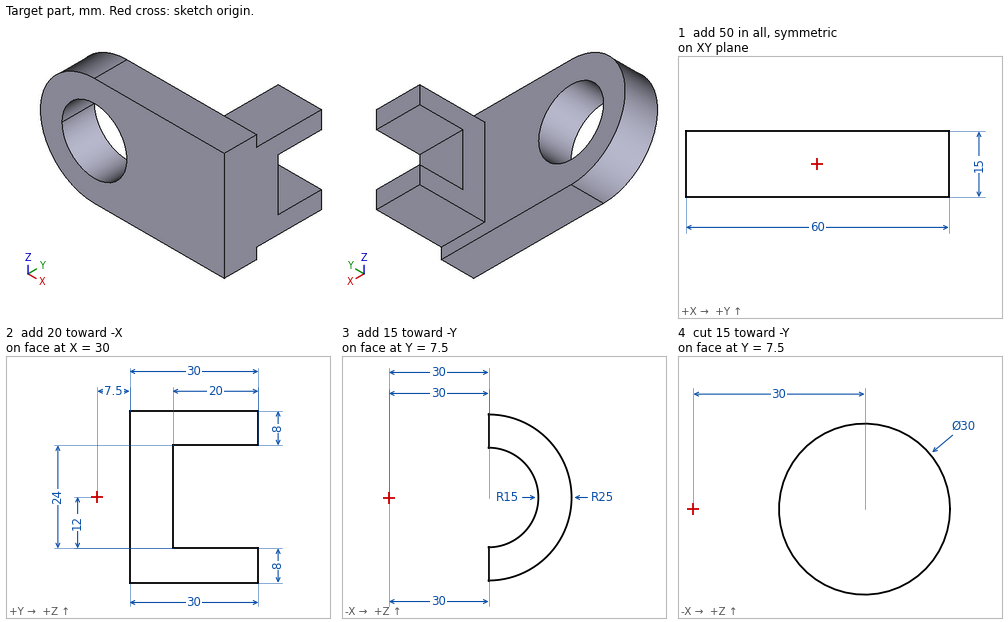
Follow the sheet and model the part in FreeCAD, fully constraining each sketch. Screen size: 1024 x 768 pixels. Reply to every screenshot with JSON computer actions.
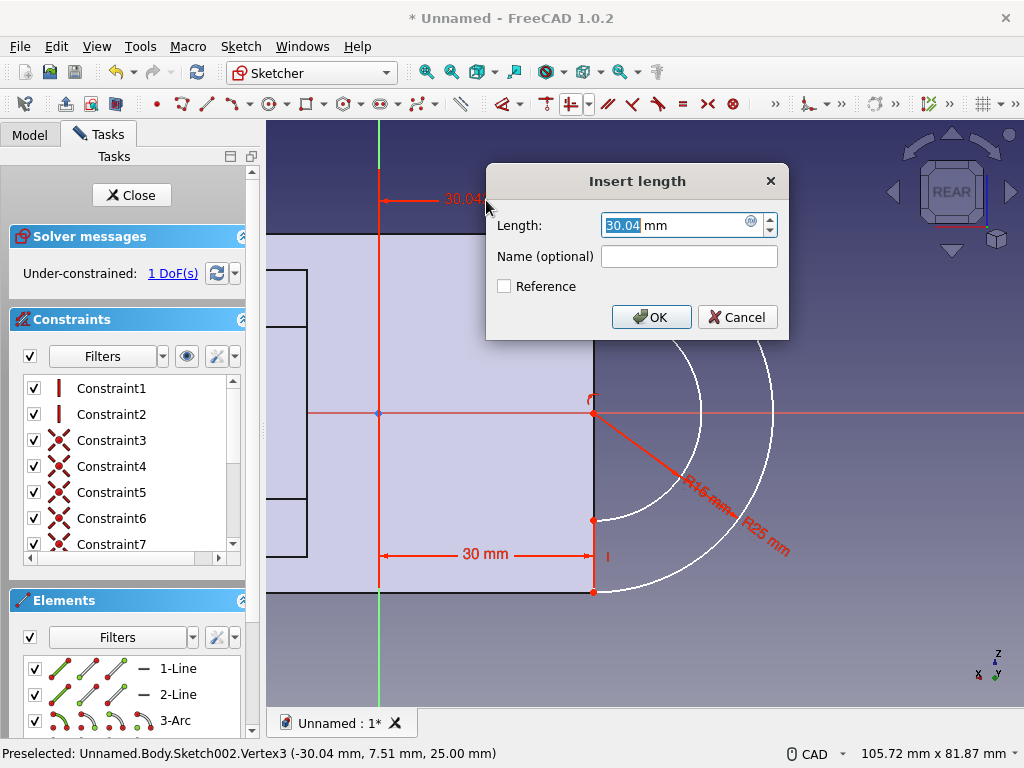
{"action": "type", "text": "30"}
{"action": "key", "text": "Return"}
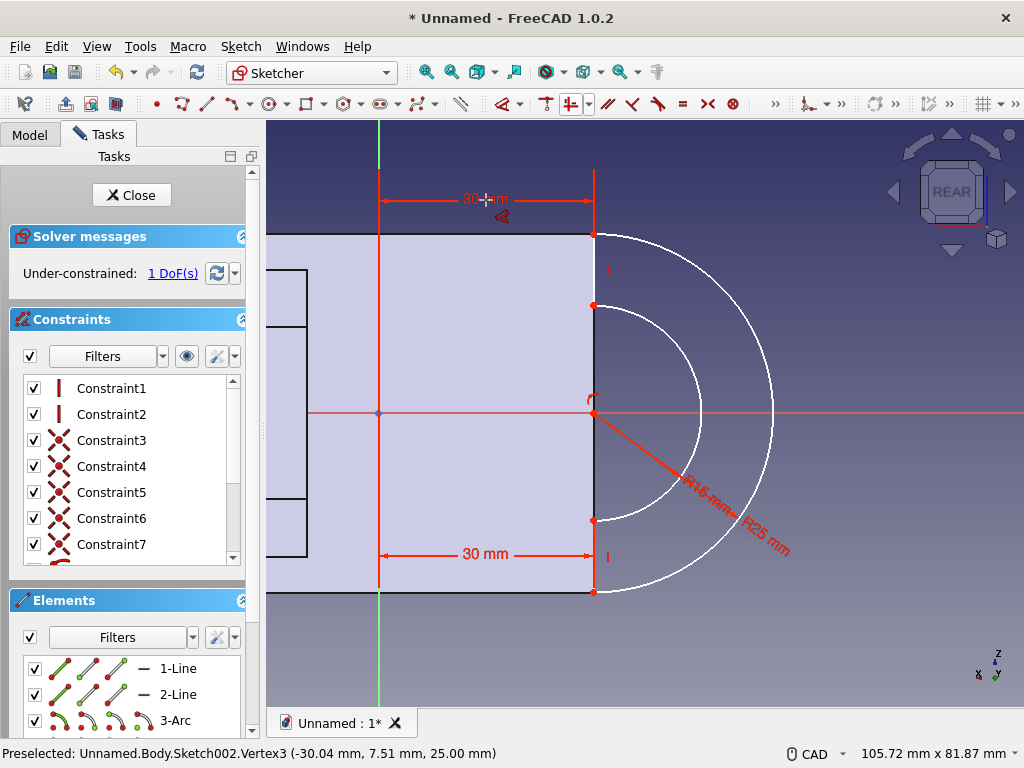
{"action": "left_click", "coordinate": [594, 413]}
{"action": "left_click", "coordinate": [486, 447]}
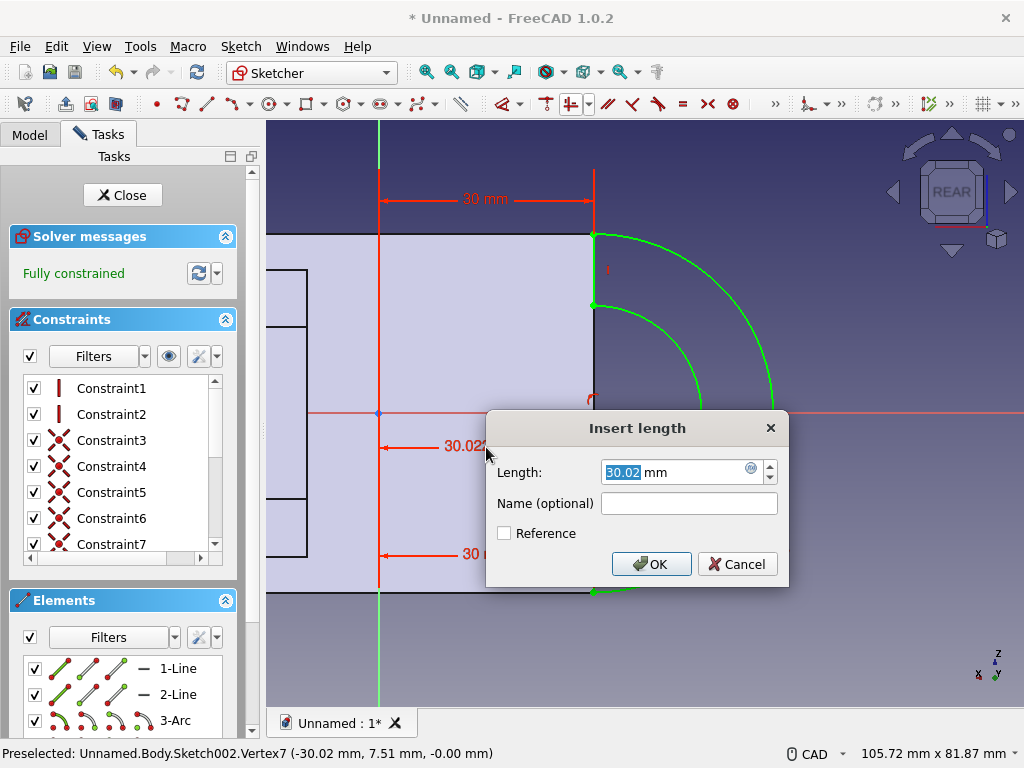
{"action": "type", "text": "30"}
{"action": "key", "text": "Return"}
{"action": "key", "text": "Escape"}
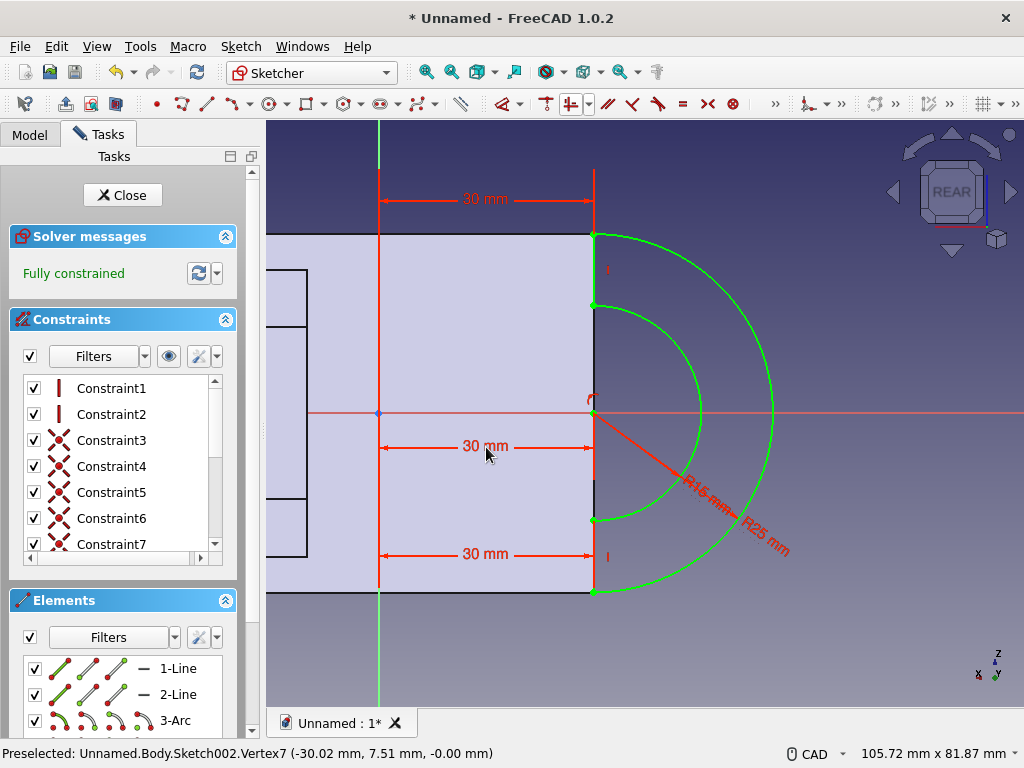
{"action": "left_click", "coordinate": [123, 195]}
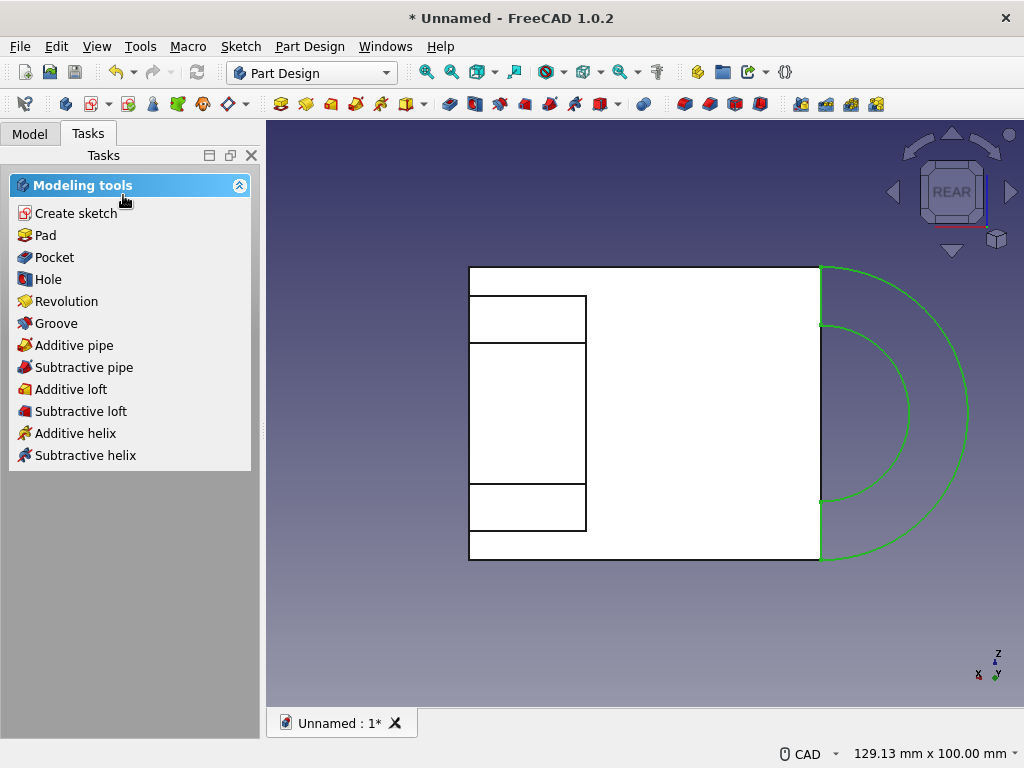
{"action": "left_click", "coordinate": [281, 104]}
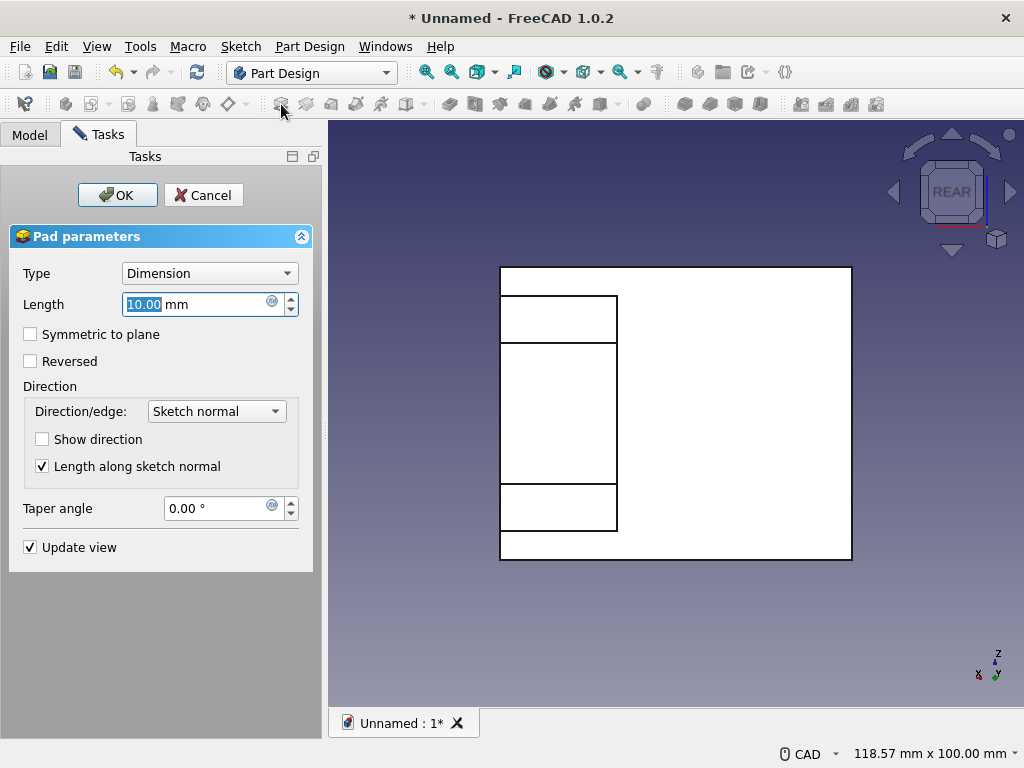
{"action": "type", "text": "15"}
{"action": "key", "text": "Tab"}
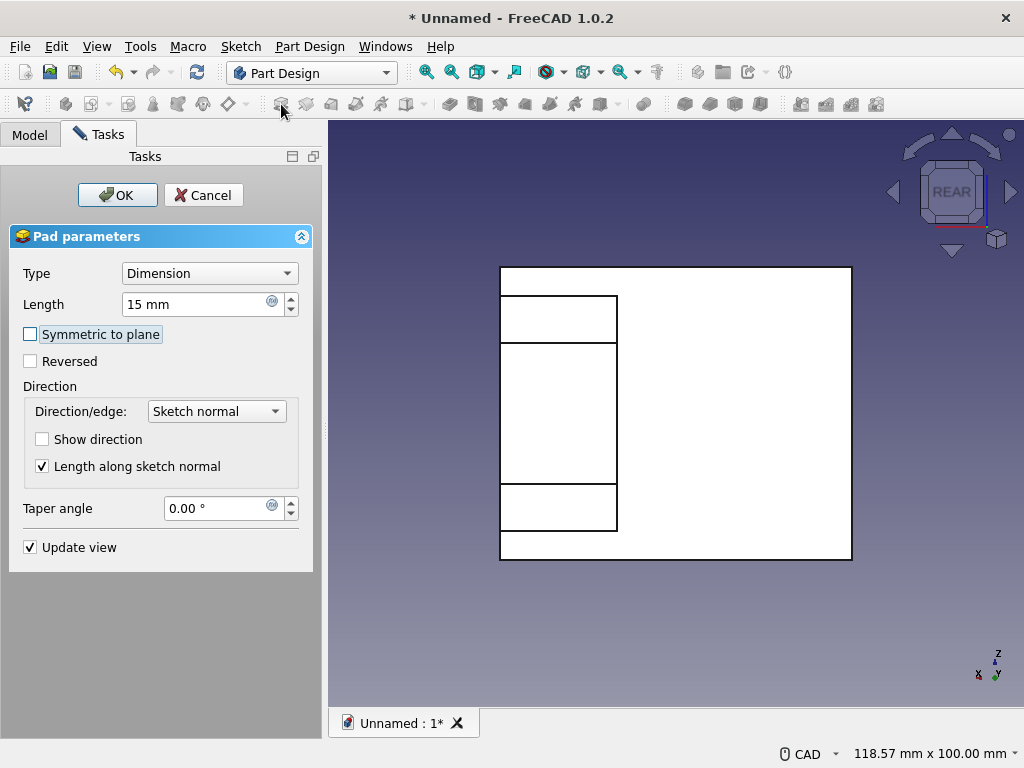
{"action": "left_click", "coordinate": [31, 361]}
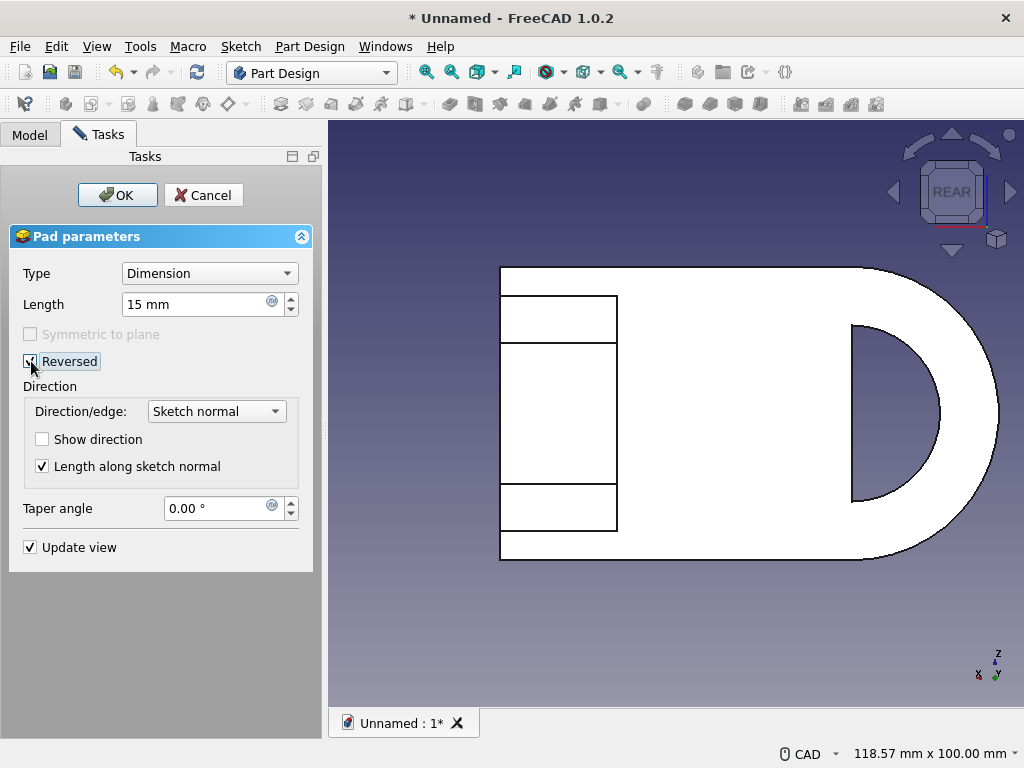
{"action": "left_click", "coordinate": [118, 195]}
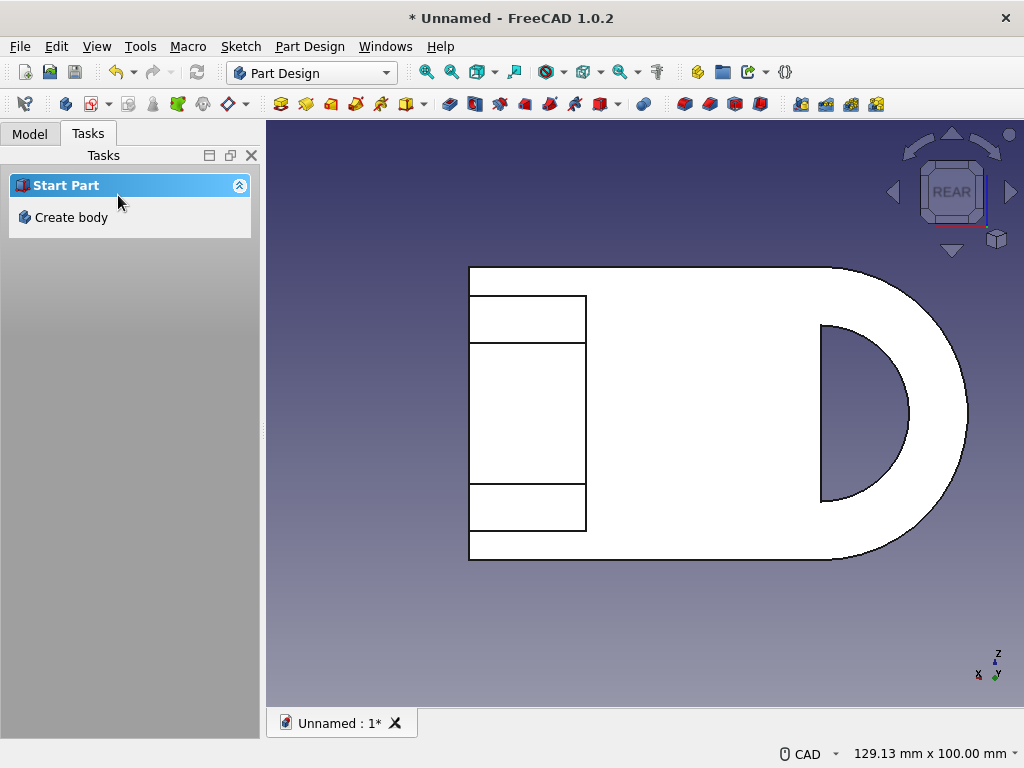
{"action": "left_click", "coordinate": [718, 371]}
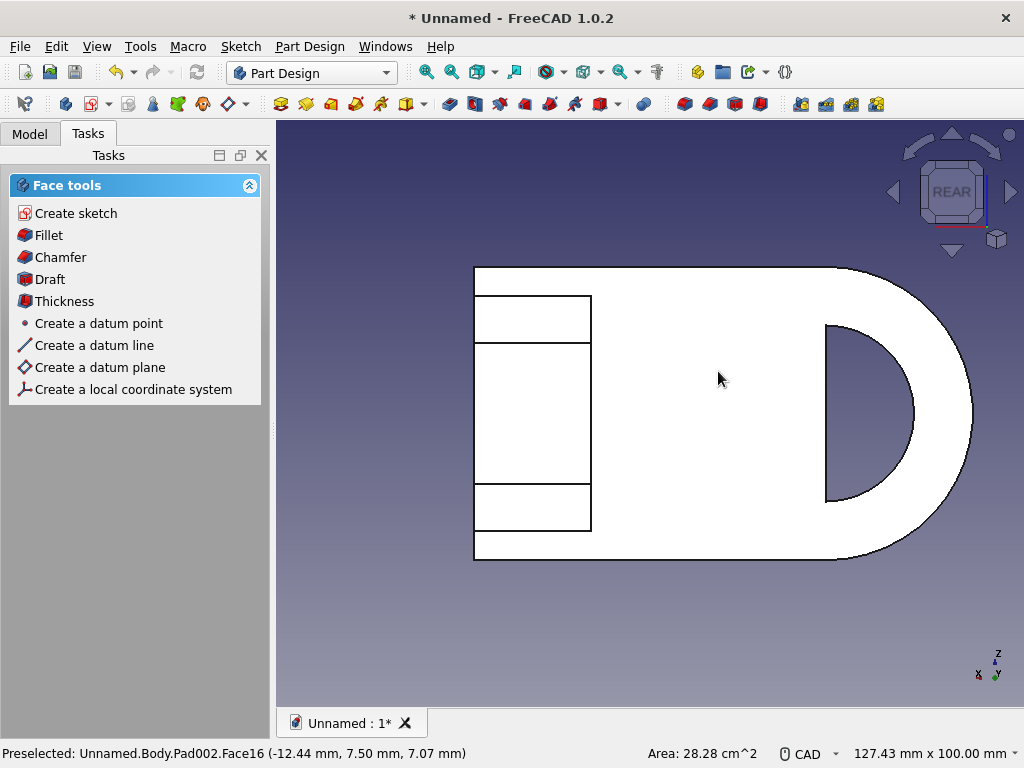
{"action": "left_click", "coordinate": [90, 104]}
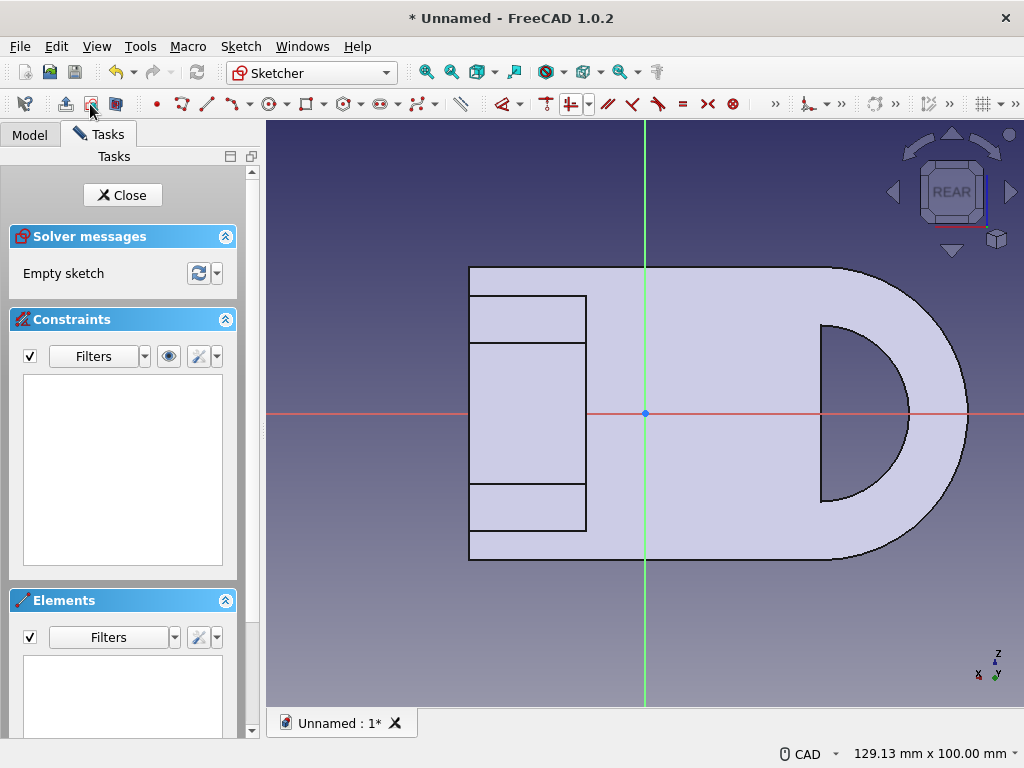
{"action": "left_click", "coordinate": [116, 104]}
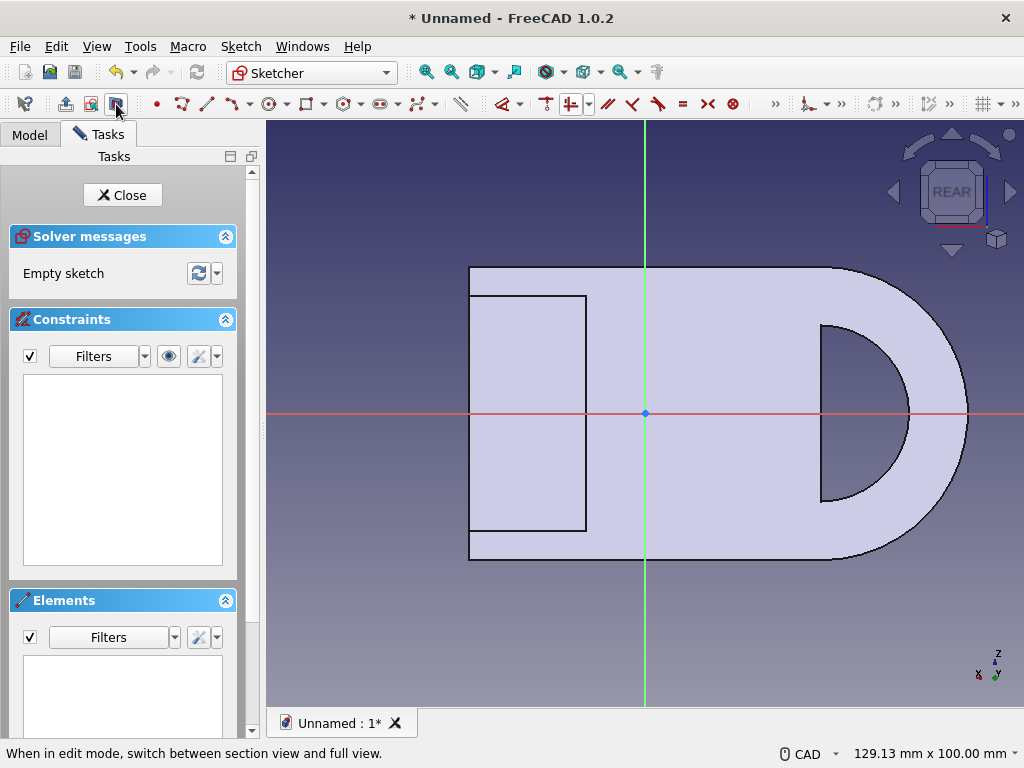
{"action": "scroll", "coordinate": [294, 413], "scroll_direction": "down", "scroll_amount": 1}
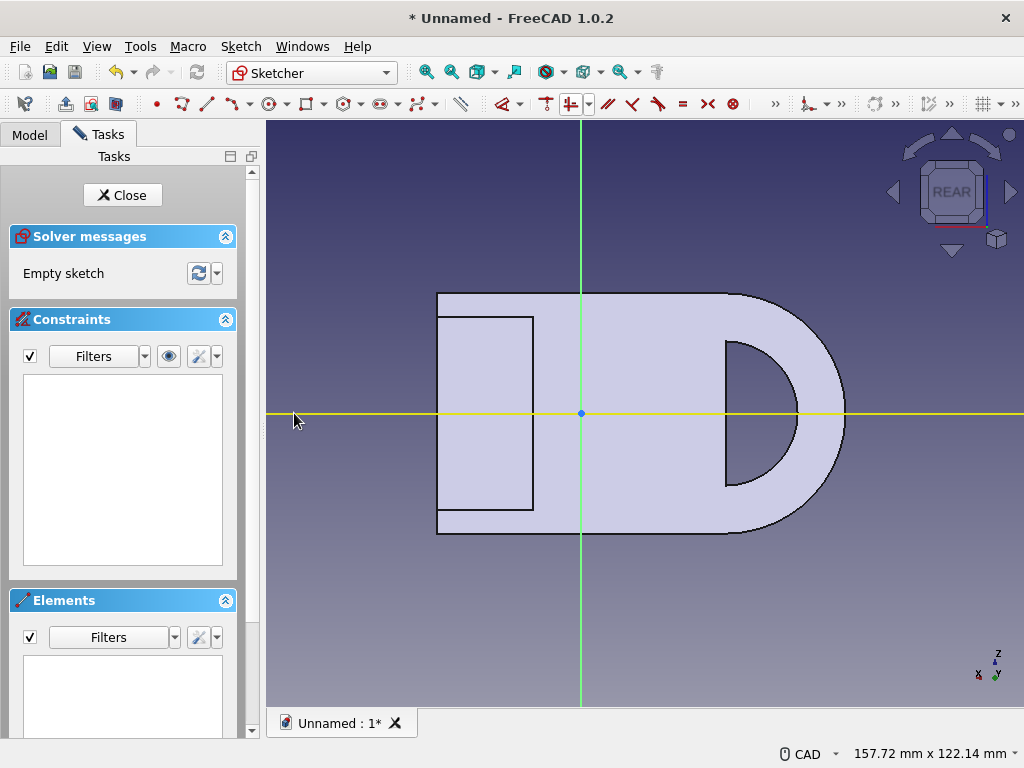
{"action": "scroll", "coordinate": [827, 414], "scroll_direction": "up", "scroll_amount": 3}